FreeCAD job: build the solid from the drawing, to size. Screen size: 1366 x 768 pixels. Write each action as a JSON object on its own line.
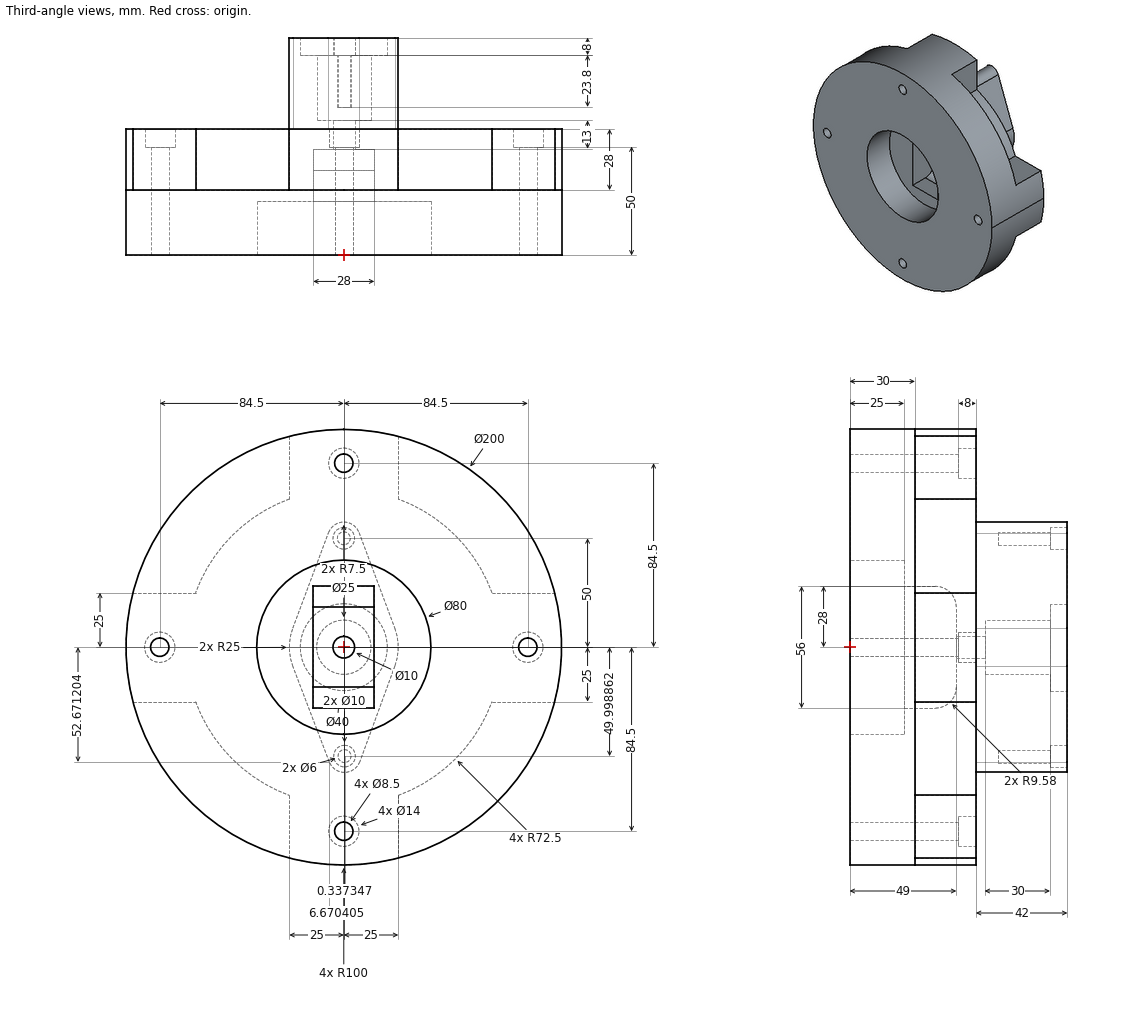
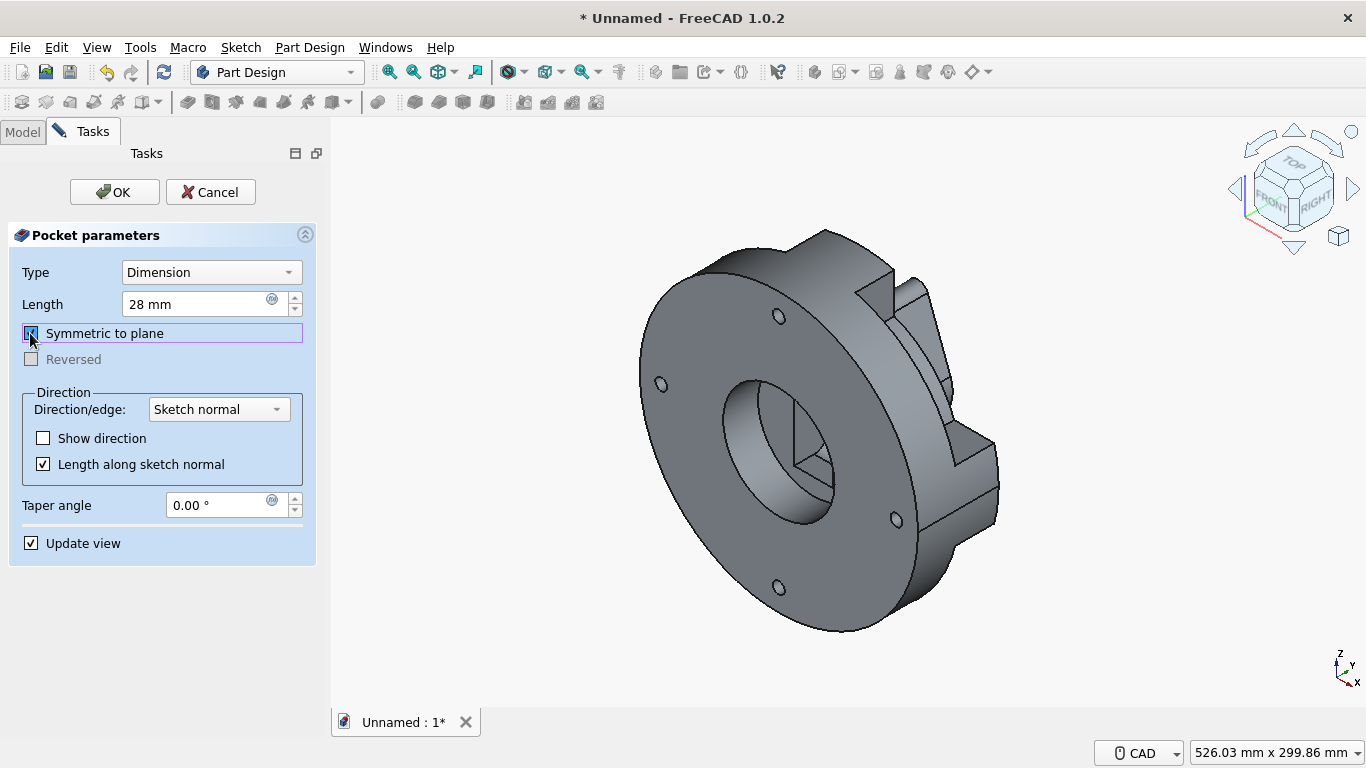
{"action": "left_click", "coordinate": [115, 192]}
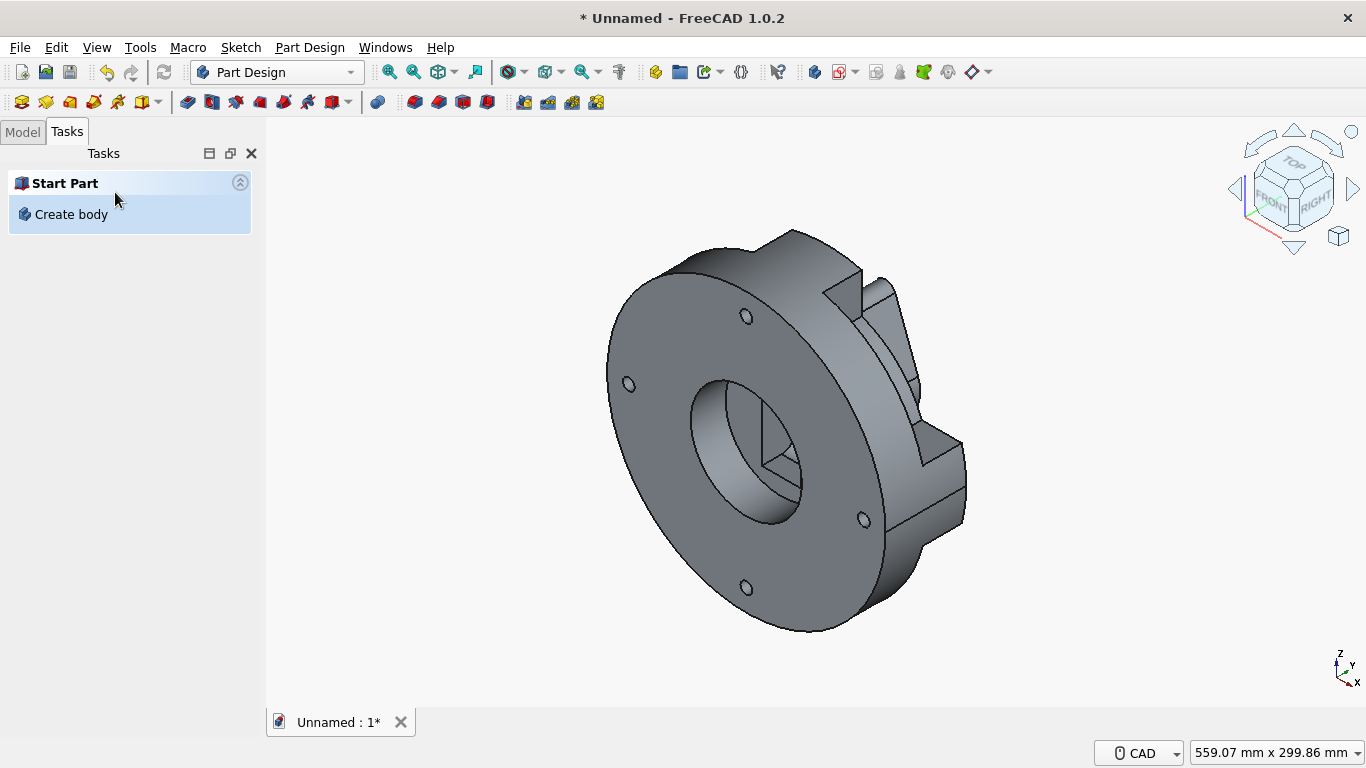
{"action": "key", "text": "4"}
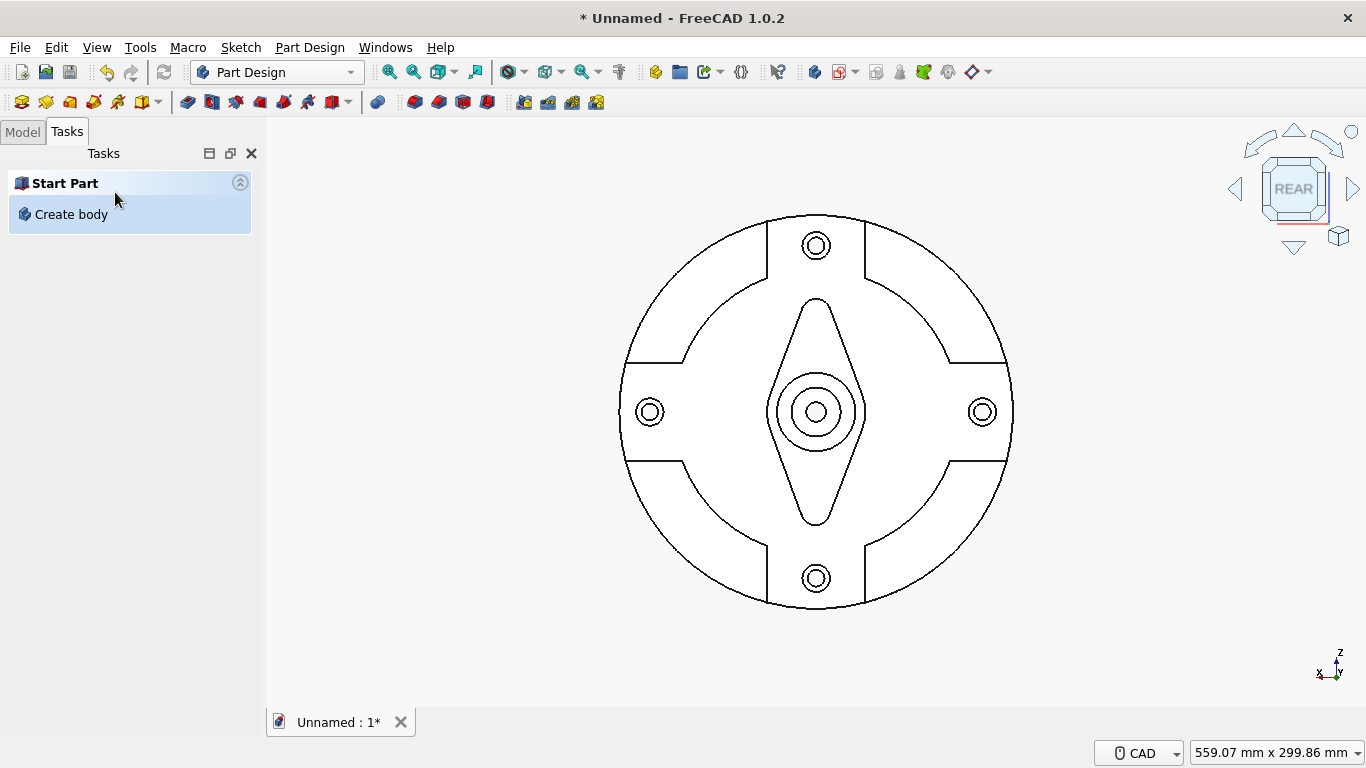
{"action": "left_click", "coordinate": [816, 346]}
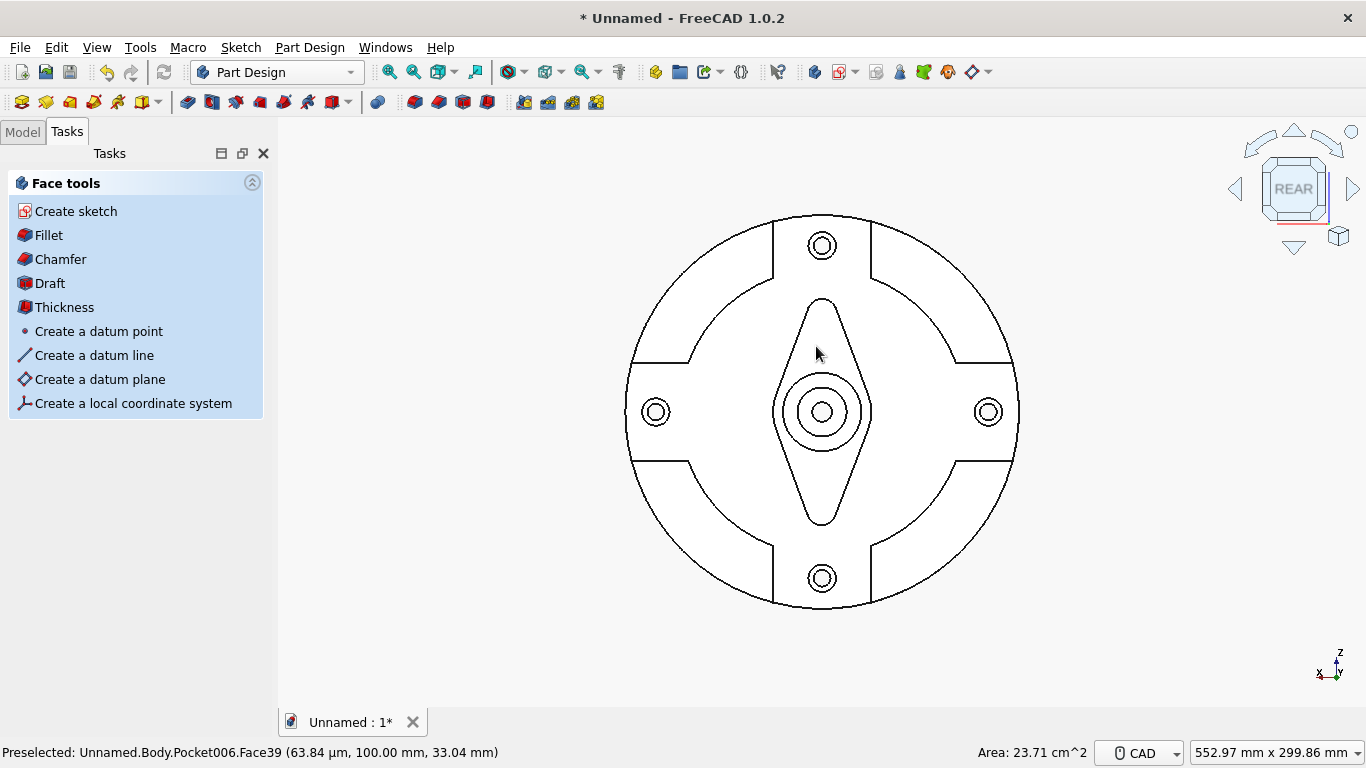
{"action": "left_click", "coordinate": [840, 72]}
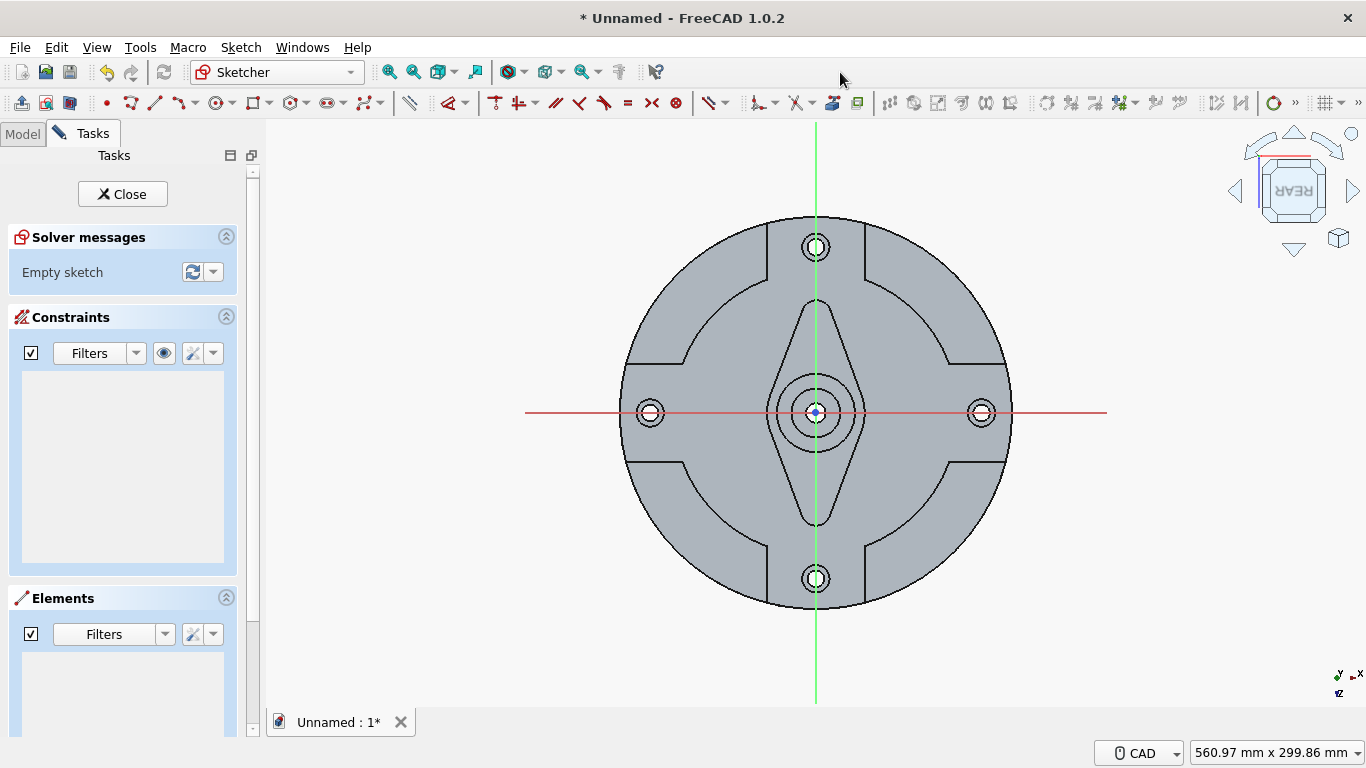
{"action": "scroll", "coordinate": [900, 413], "scroll_direction": "up", "scroll_amount": 3}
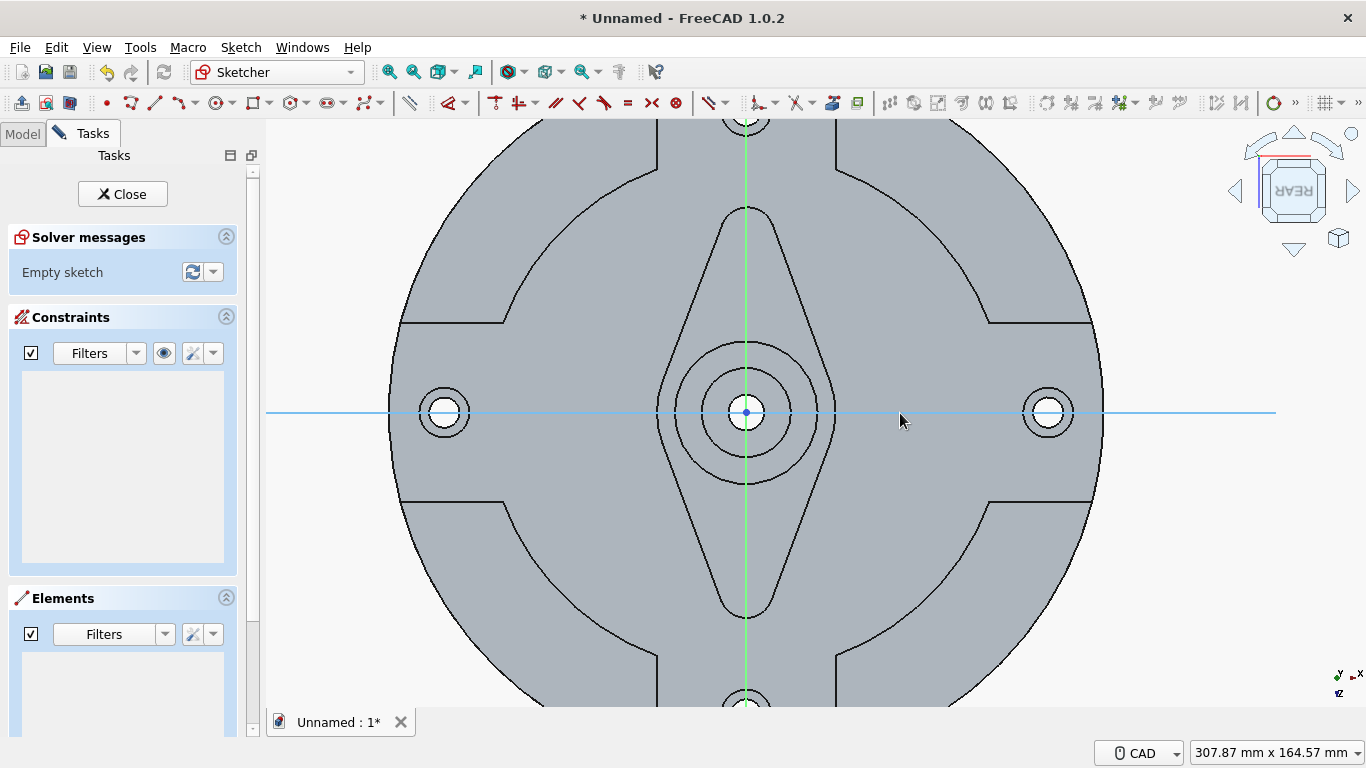
{"action": "key", "text": "g c"}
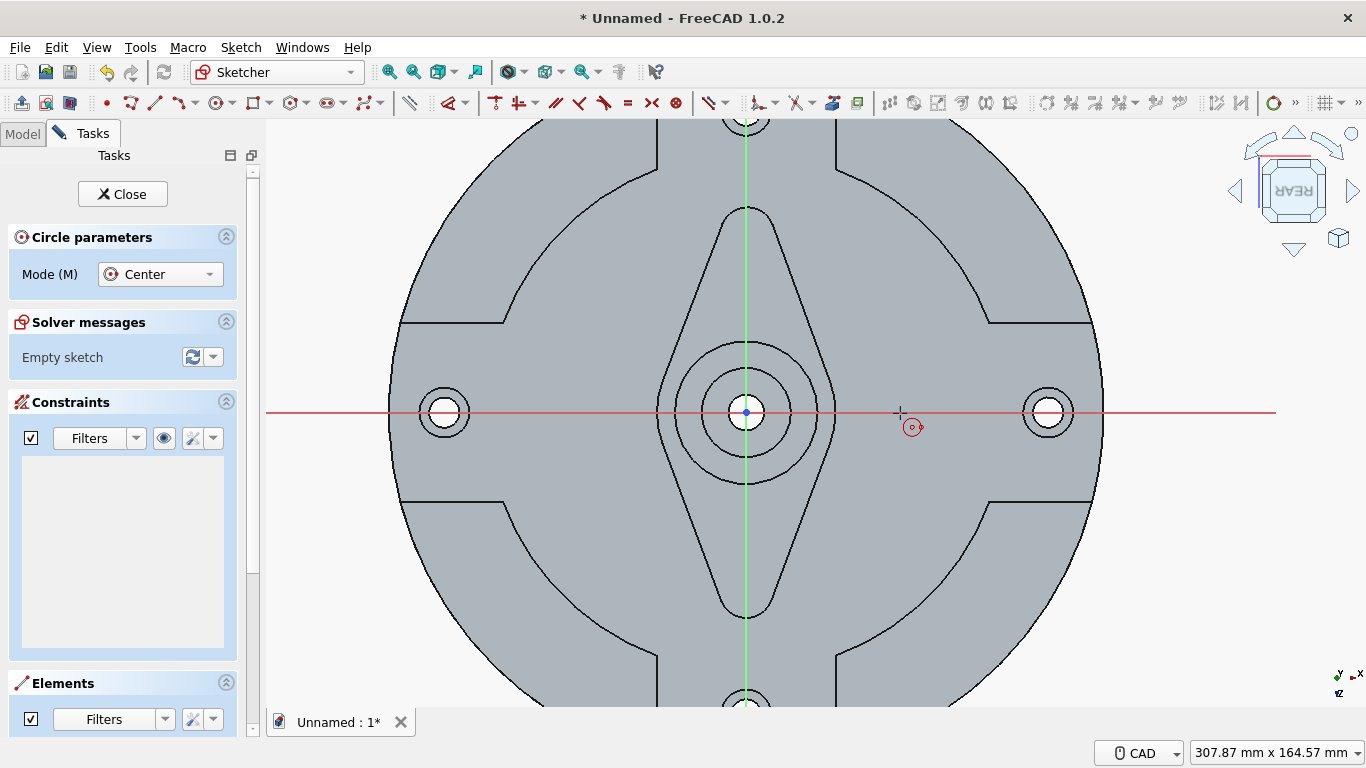
{"action": "scroll", "coordinate": [747, 234], "scroll_direction": "up", "scroll_amount": 13}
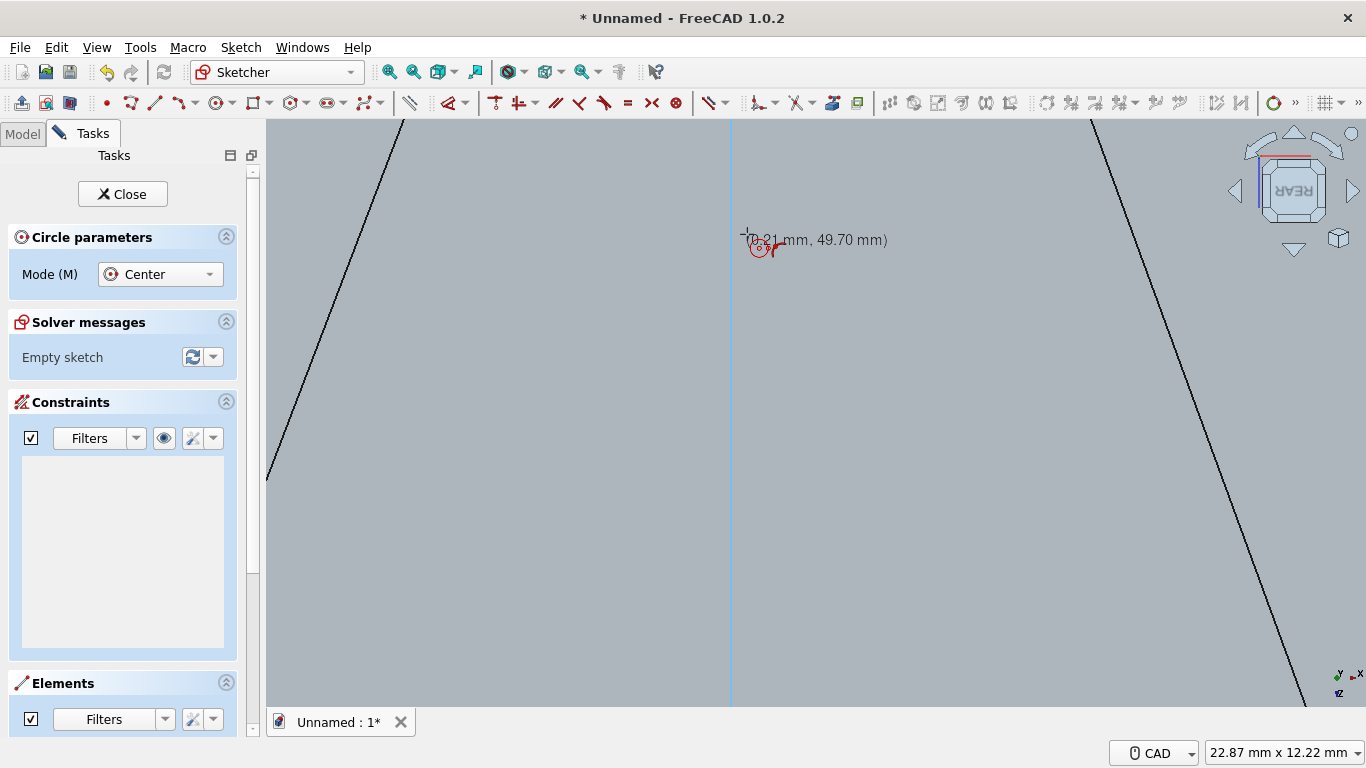
{"action": "left_click", "coordinate": [748, 231]}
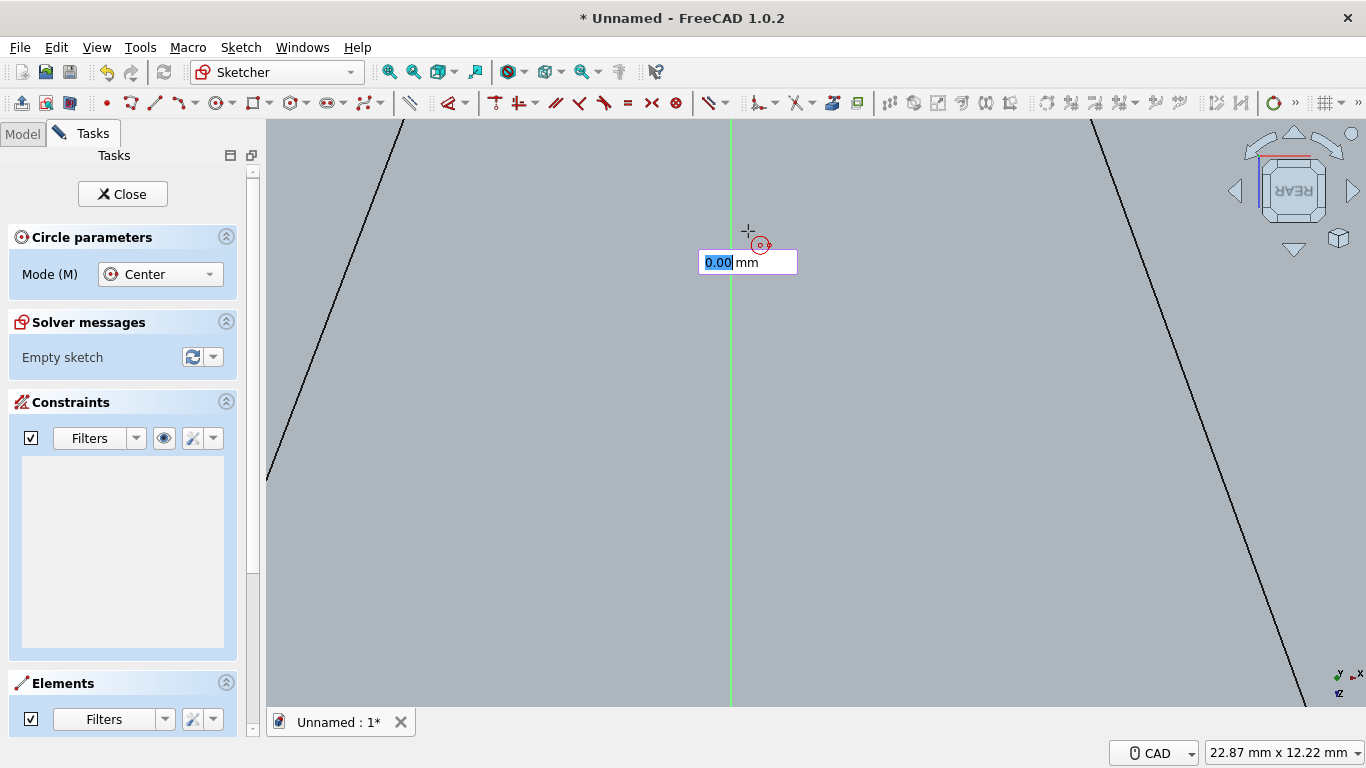
{"action": "scroll", "coordinate": [748, 235], "scroll_direction": "down", "scroll_amount": 13}